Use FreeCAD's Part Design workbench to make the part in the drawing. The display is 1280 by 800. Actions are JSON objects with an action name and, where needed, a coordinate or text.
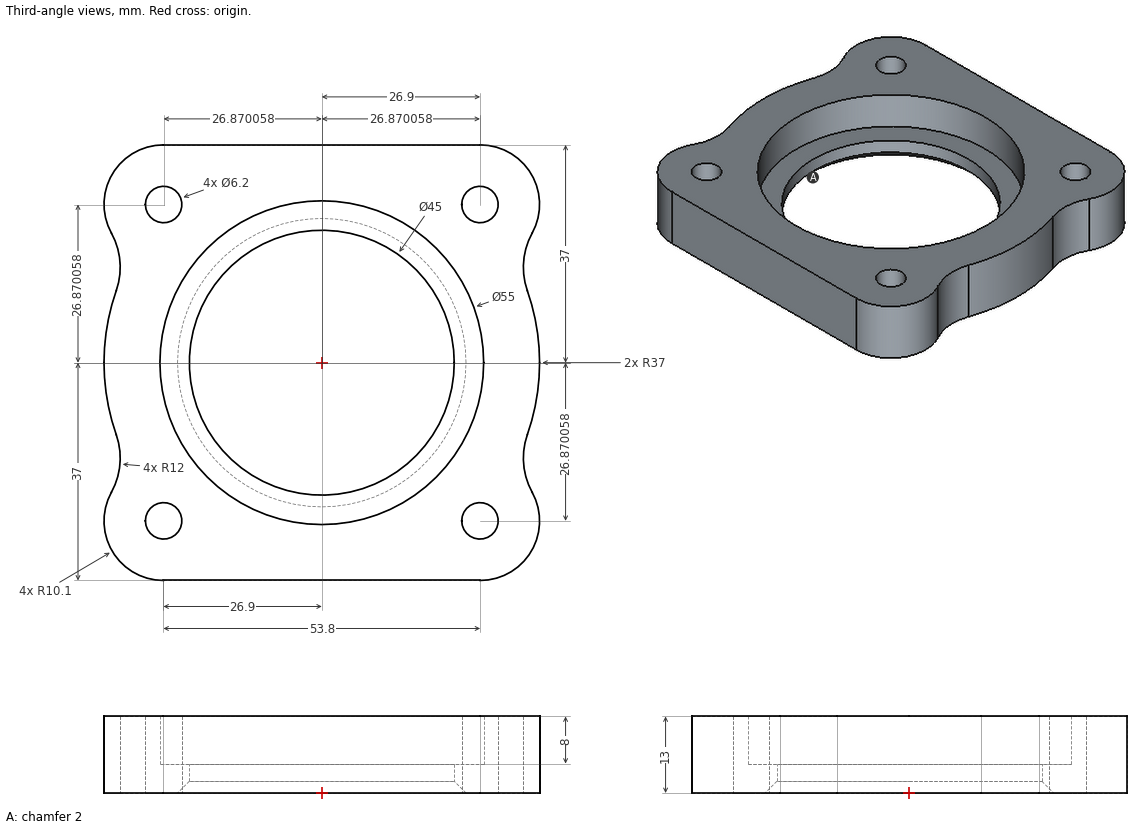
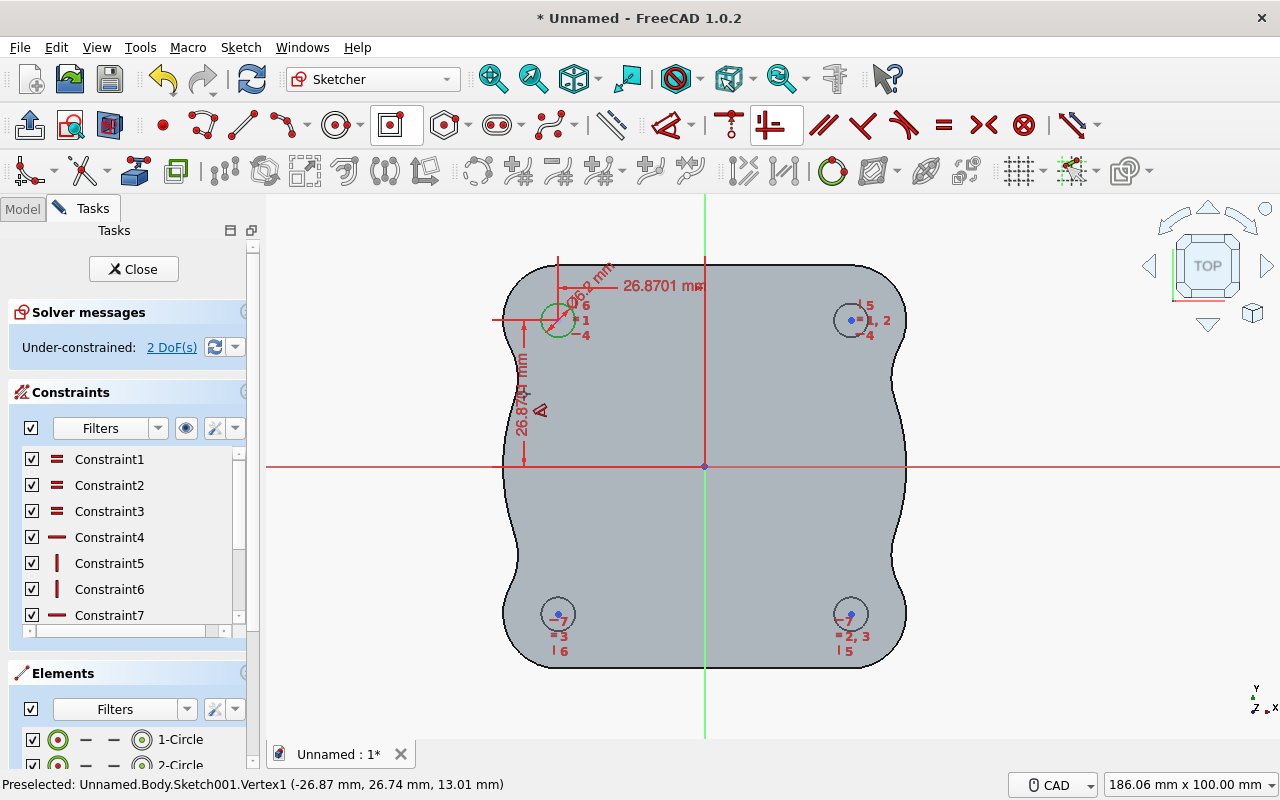
{"action": "left_click", "coordinate": [851, 320]}
{"action": "left_click", "coordinate": [778, 286]}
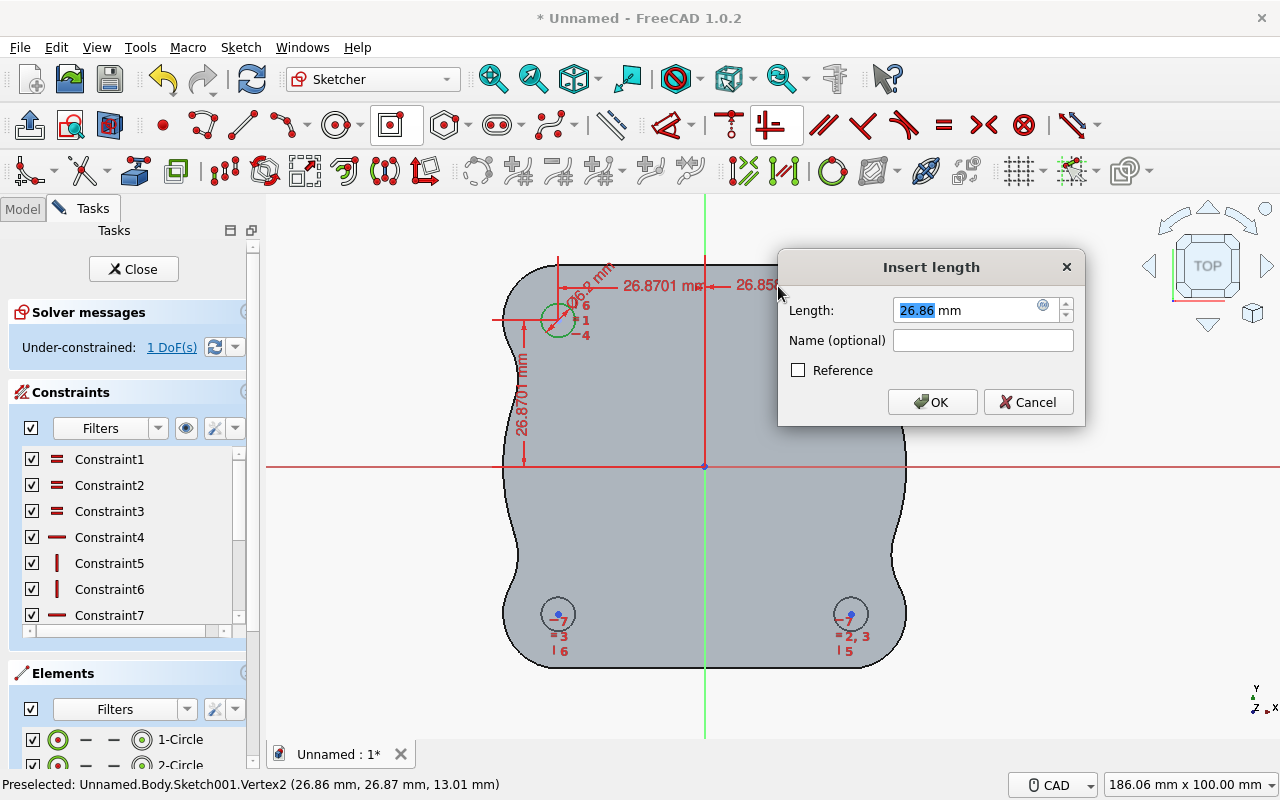
{"action": "type", "text": "26.870058"}
{"action": "key", "text": "Return"}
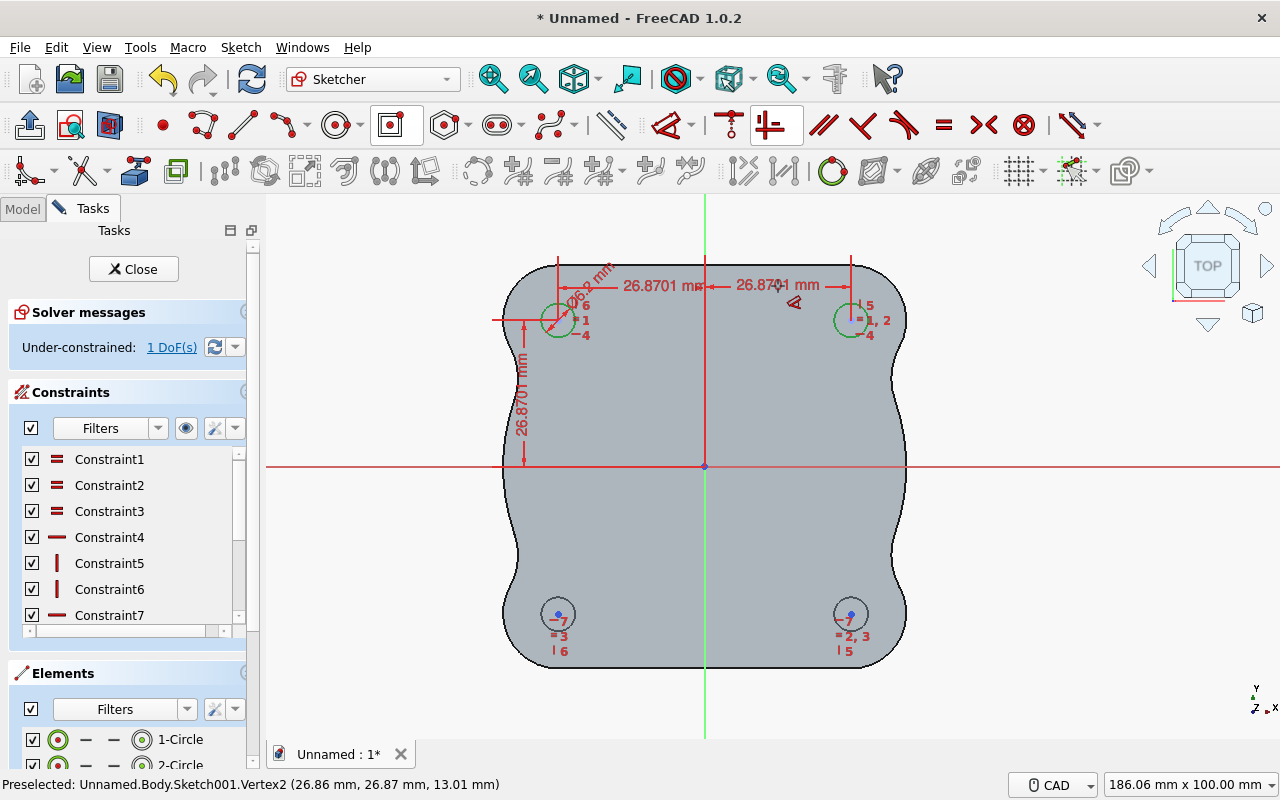
{"action": "left_click", "coordinate": [851, 614]}
{"action": "left_click", "coordinate": [885, 541]}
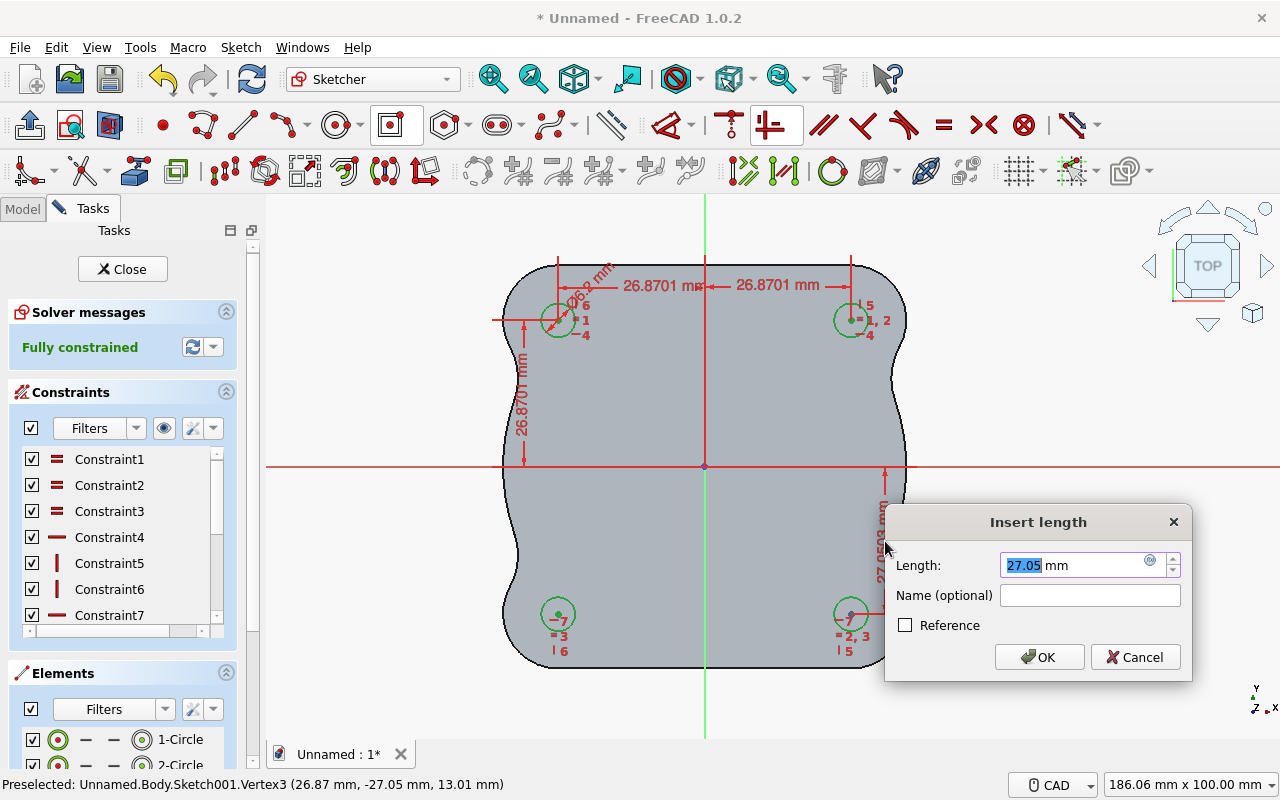
{"action": "type", "text": "26.870058"}
{"action": "key", "text": "Return"}
{"action": "key", "text": "Escape"}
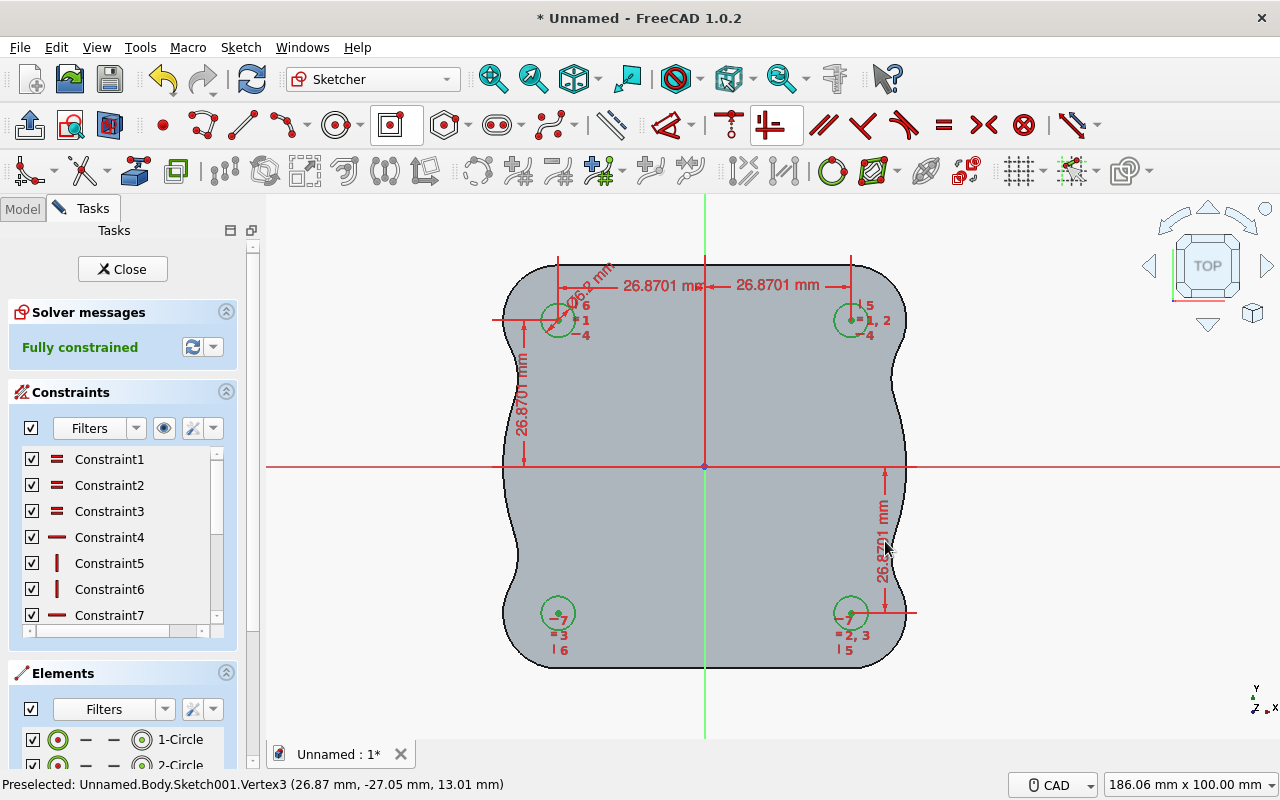
{"action": "left_click", "coordinate": [123, 269]}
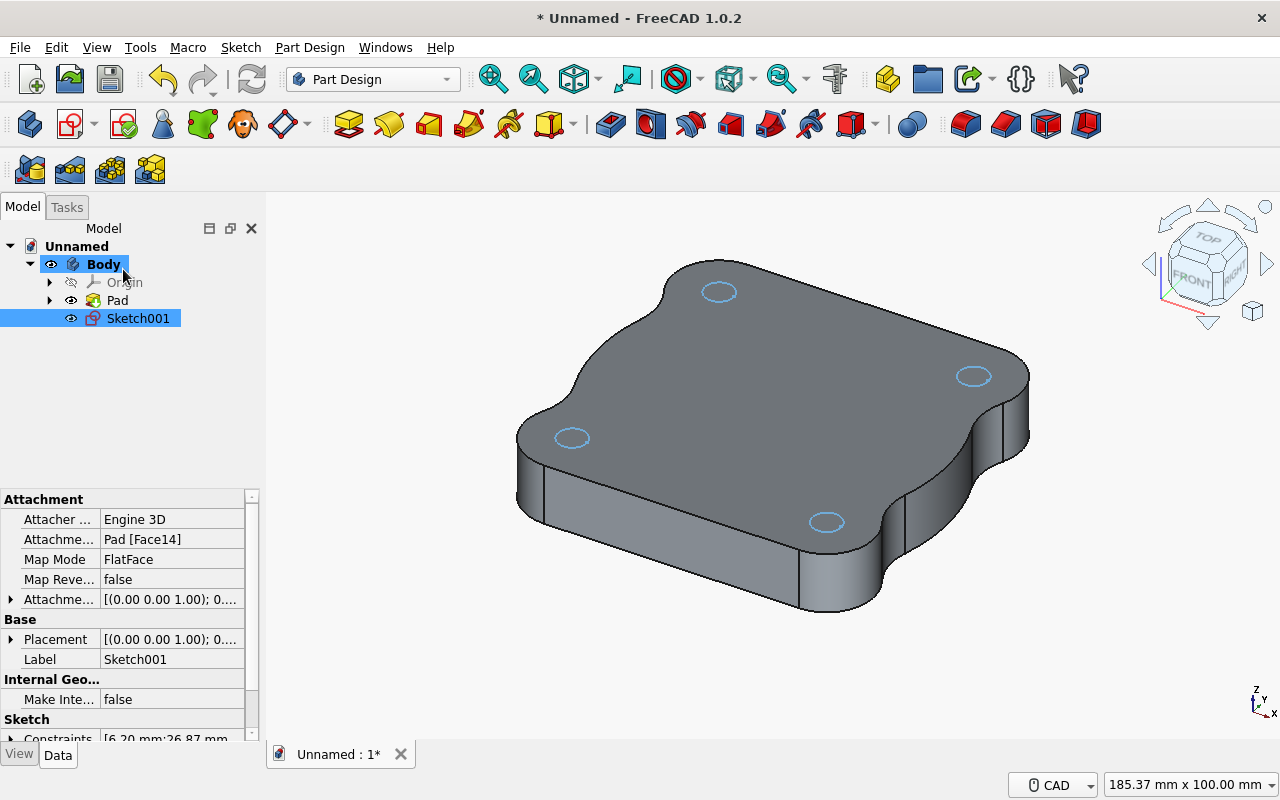
{"action": "left_click", "coordinate": [612, 124]}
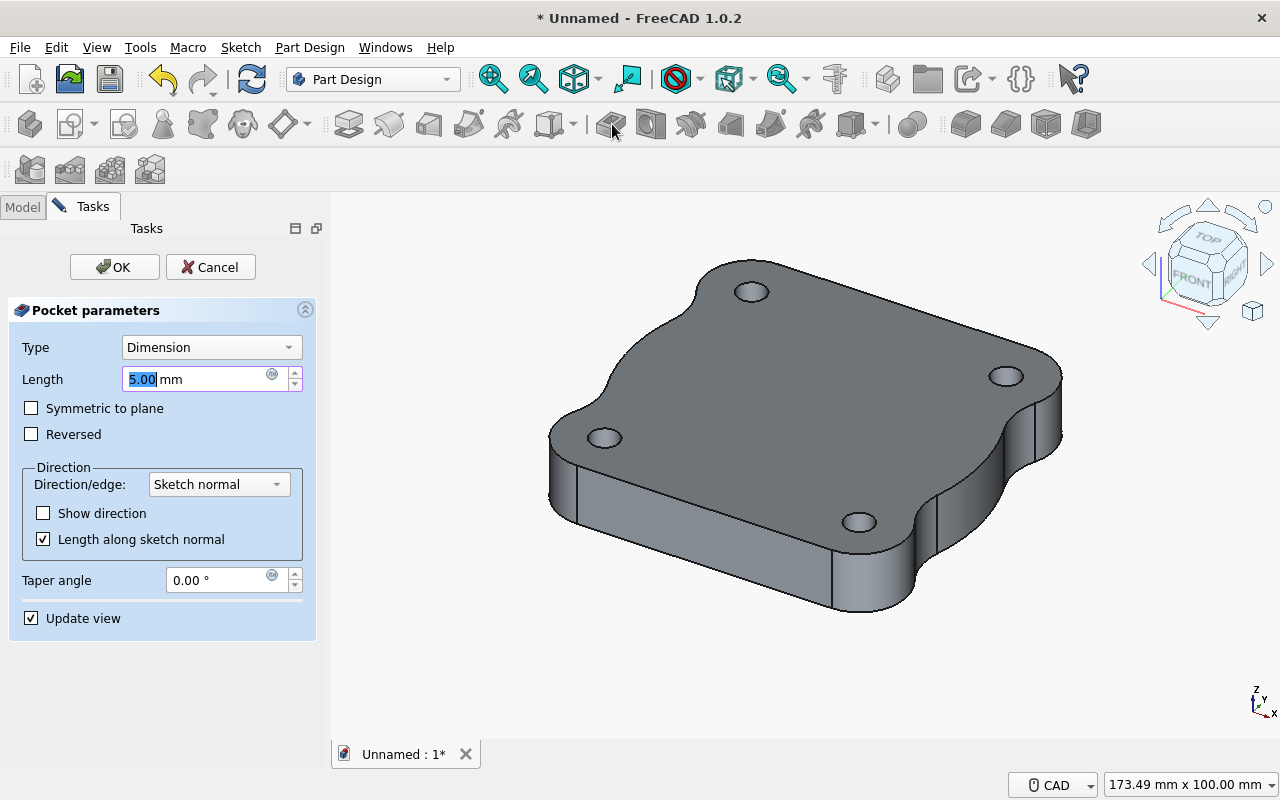
{"action": "left_click", "coordinate": [212, 348]}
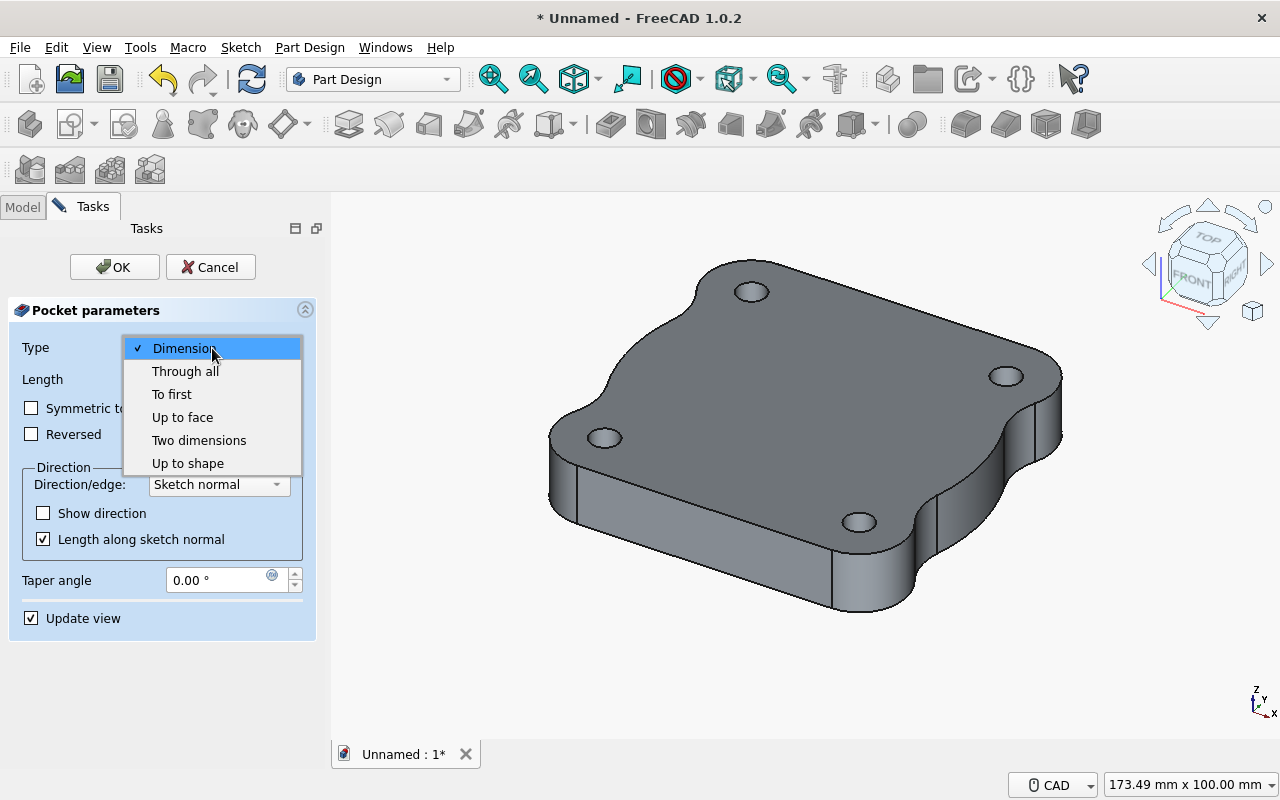
{"action": "left_click", "coordinate": [212, 372]}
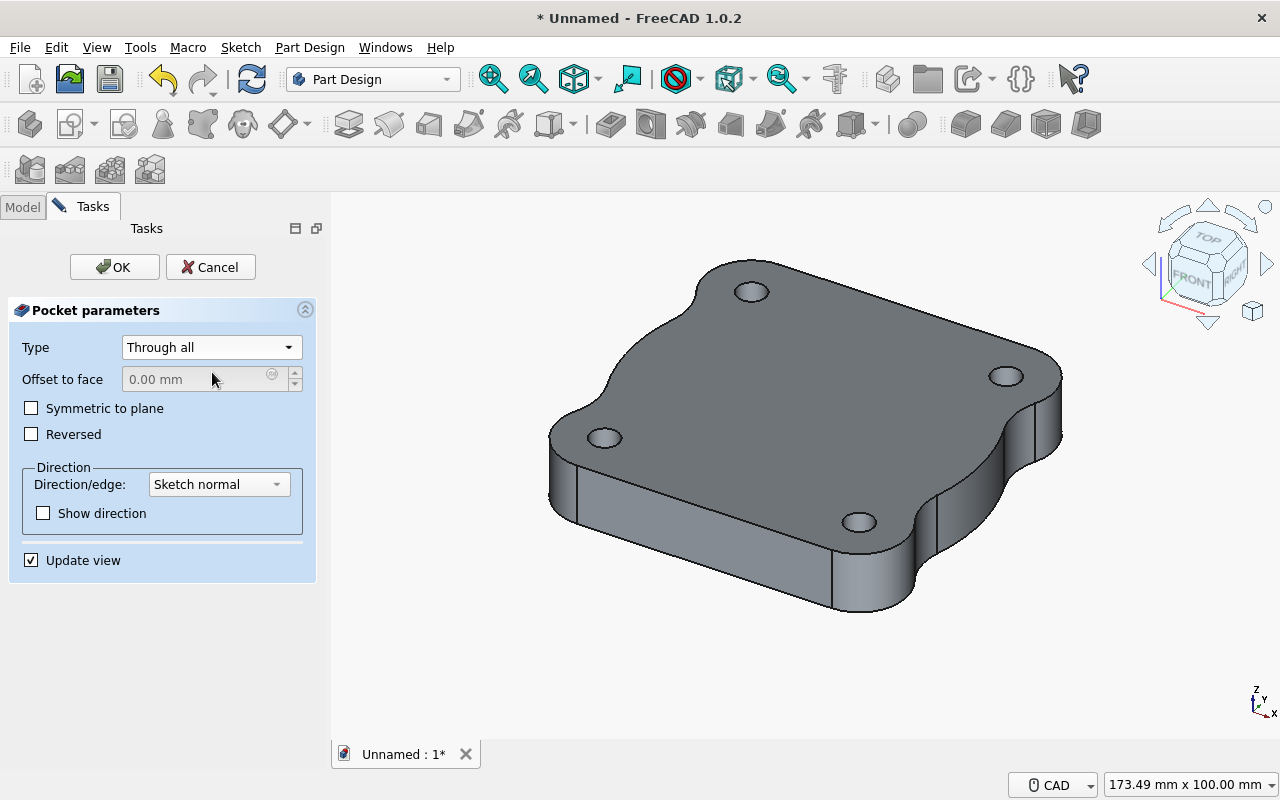
{"action": "left_click", "coordinate": [115, 267]}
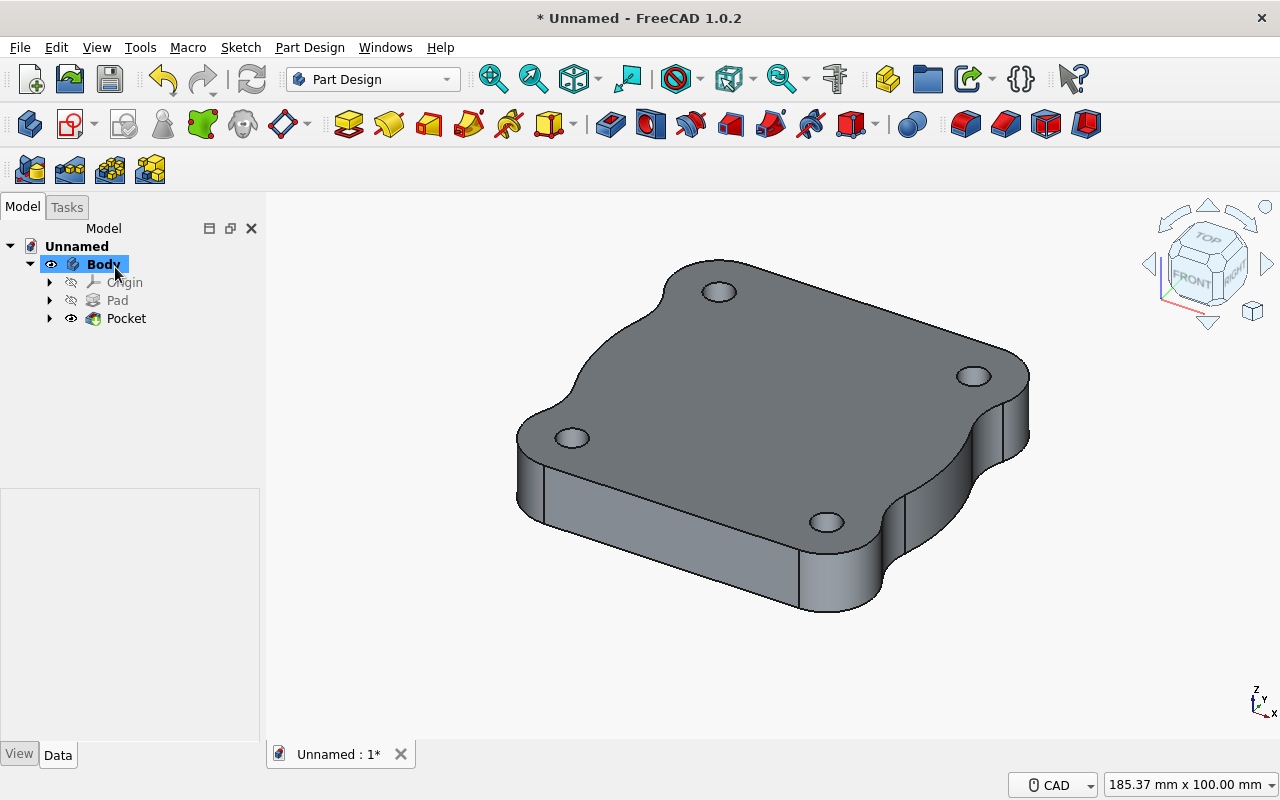
{"action": "left_click", "coordinate": [773, 406]}